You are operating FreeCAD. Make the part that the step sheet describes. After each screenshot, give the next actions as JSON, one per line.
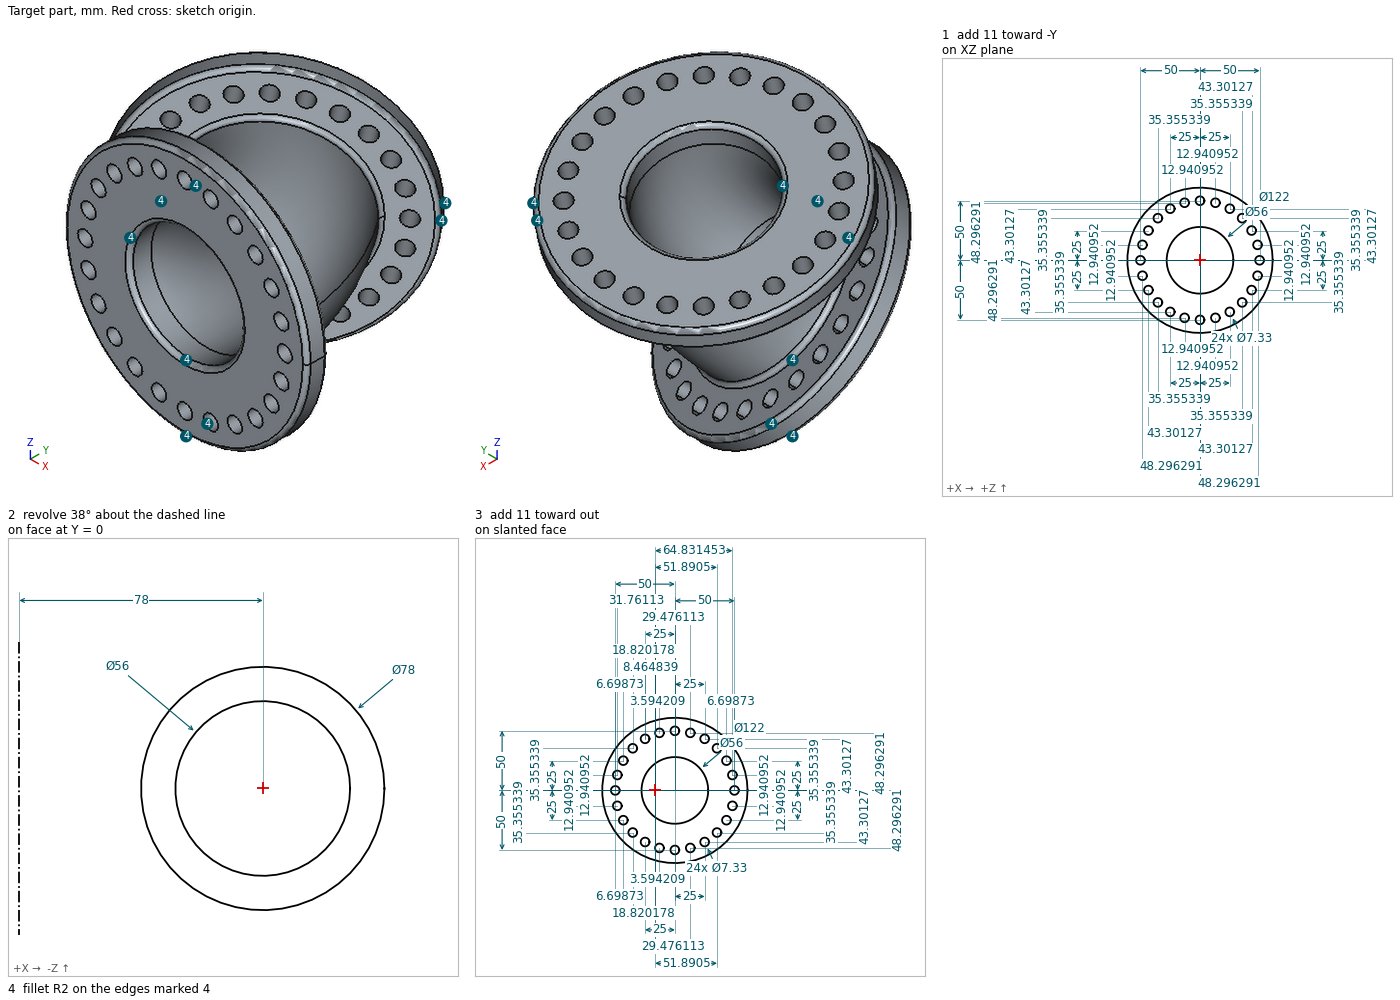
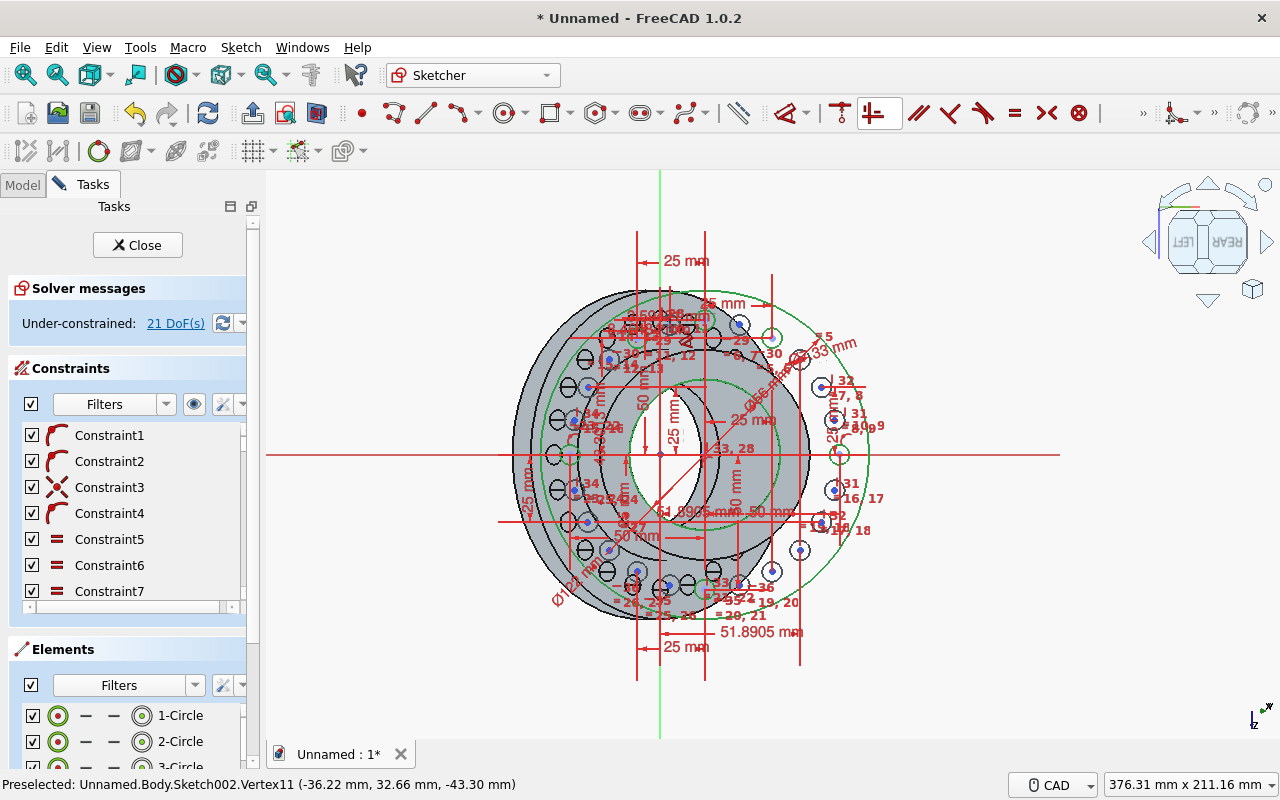
{"action": "left_click", "coordinate": [575, 420]}
{"action": "left_click", "coordinate": [637, 362]}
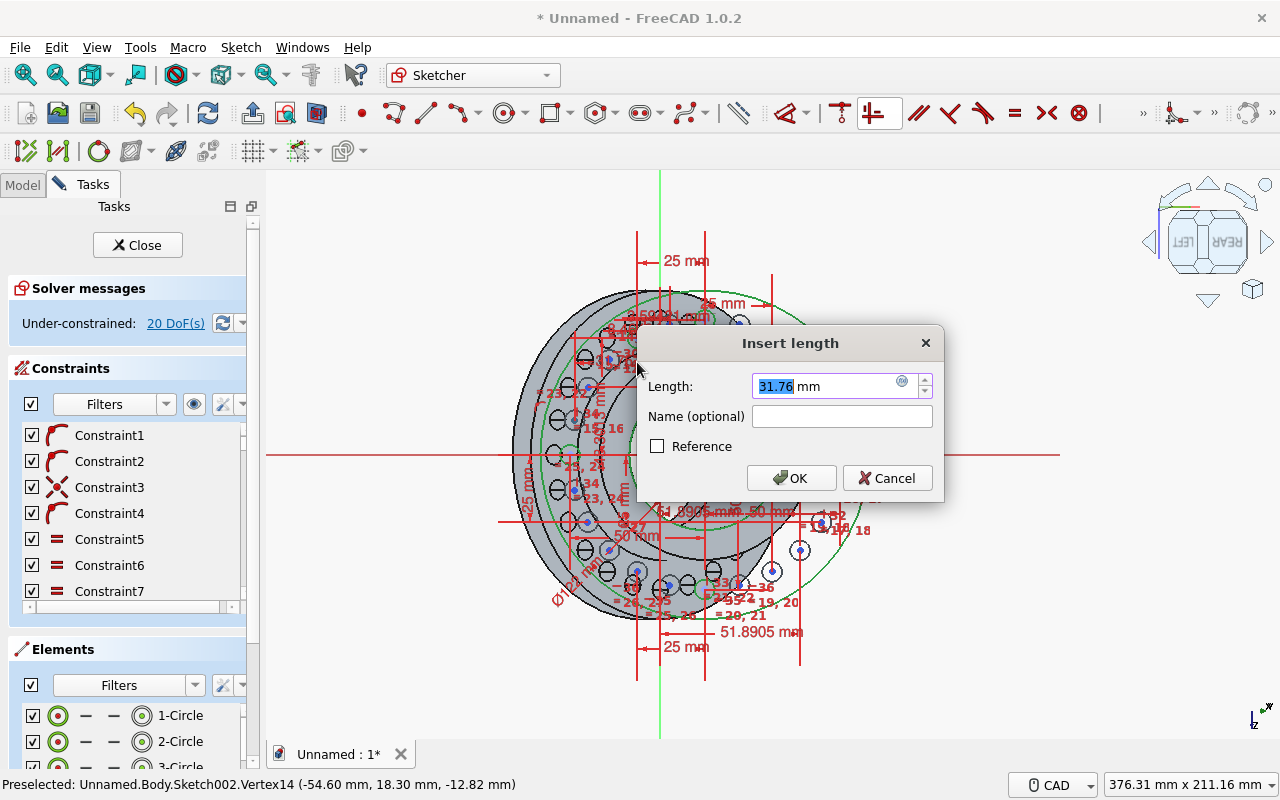
{"action": "type", "text": "31.76113"}
{"action": "key", "text": "Return"}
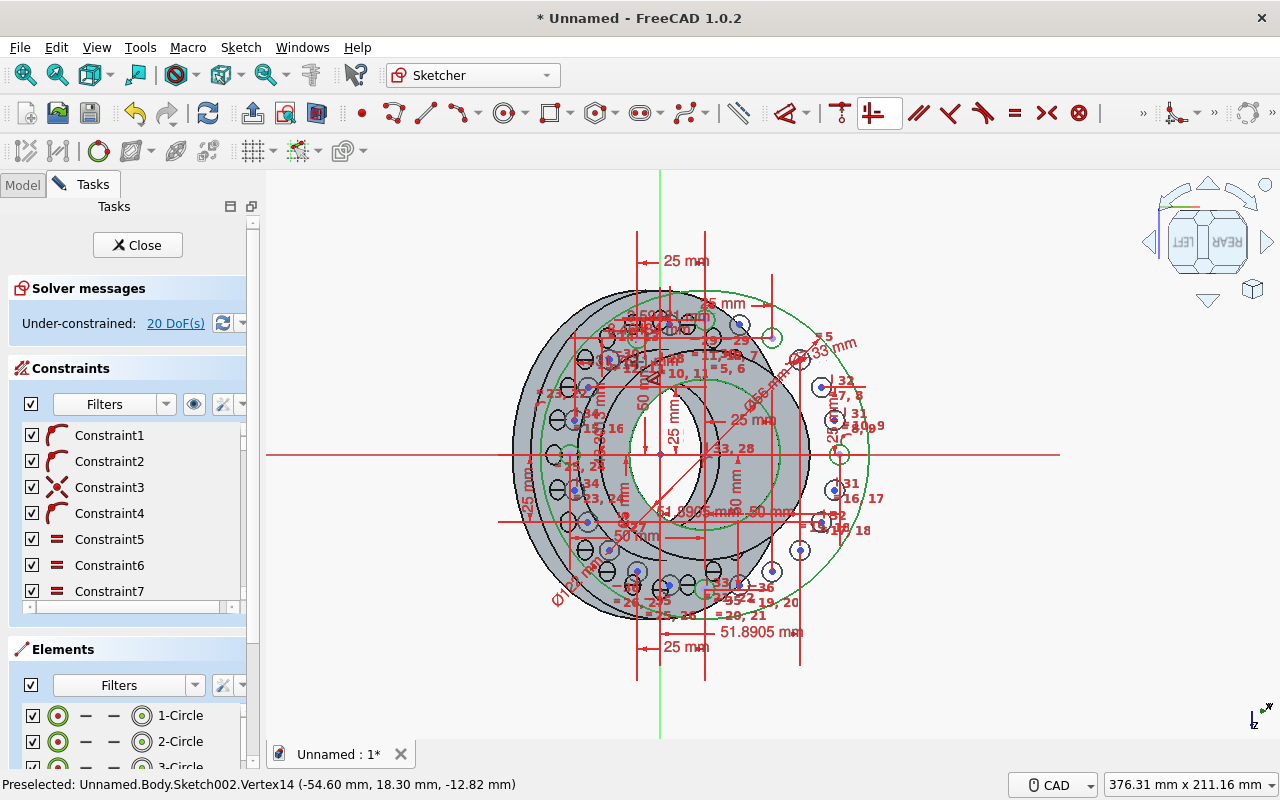
{"action": "left_click", "coordinate": [772, 572]}
{"action": "left_click", "coordinate": [602, 472]}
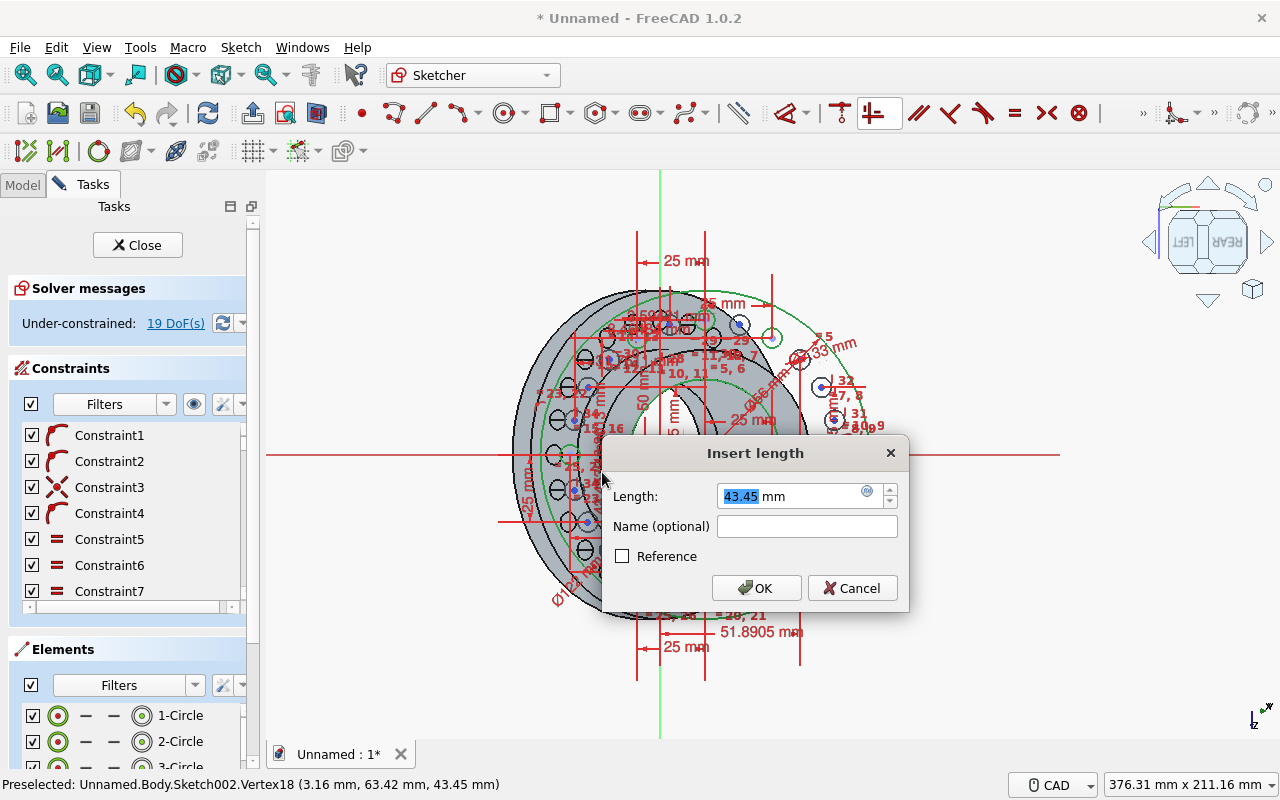
{"action": "type", "text": "43.30127"}
{"action": "key", "text": "Return"}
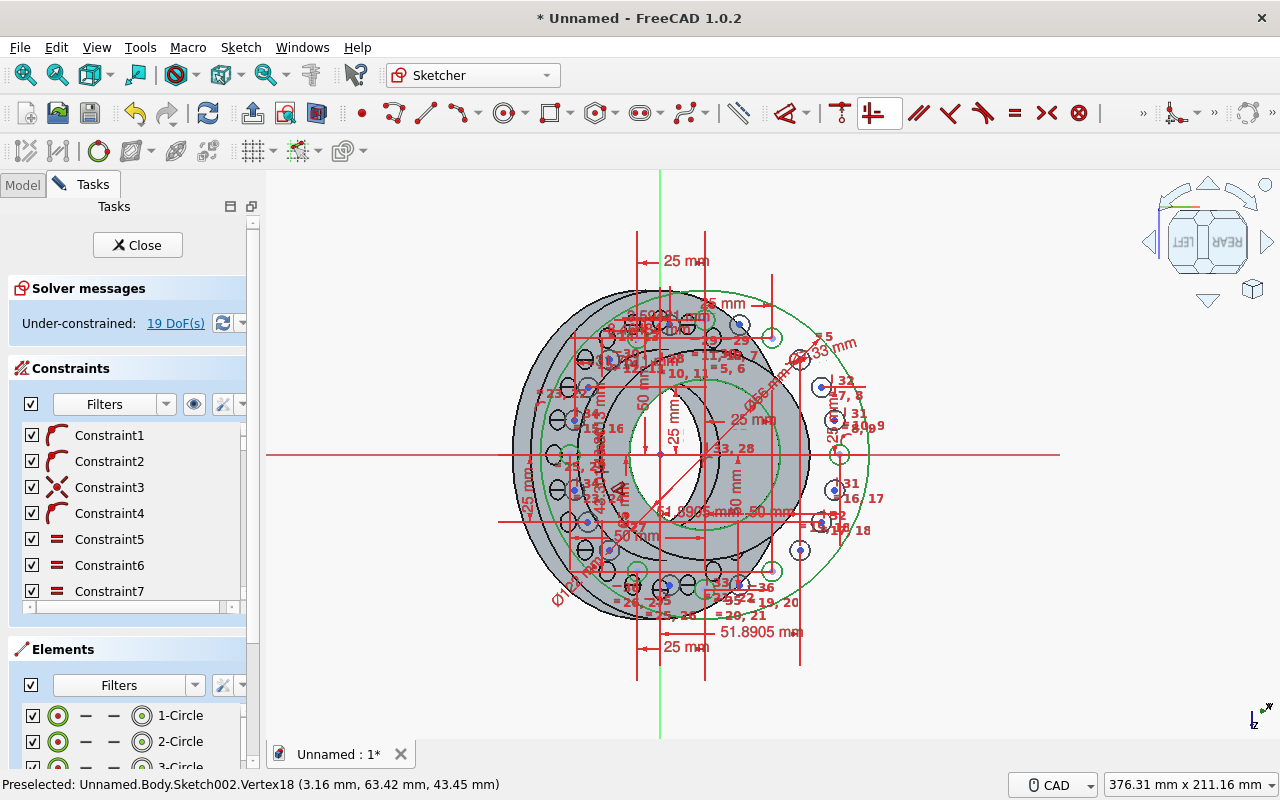
{"action": "scroll", "coordinate": [670, 585], "scroll_direction": "up", "scroll_amount": 8}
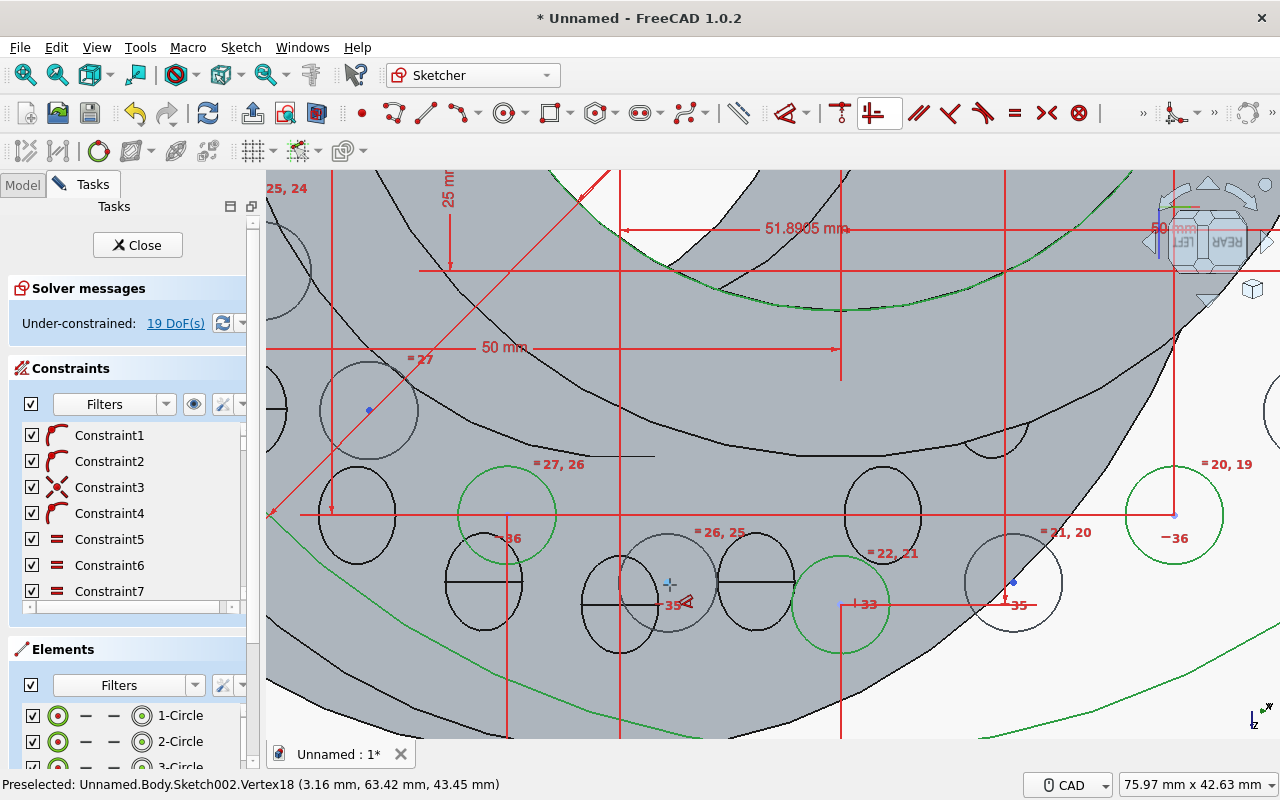
{"action": "left_click", "coordinate": [668, 583]}
{"action": "left_click", "coordinate": [661, 617]}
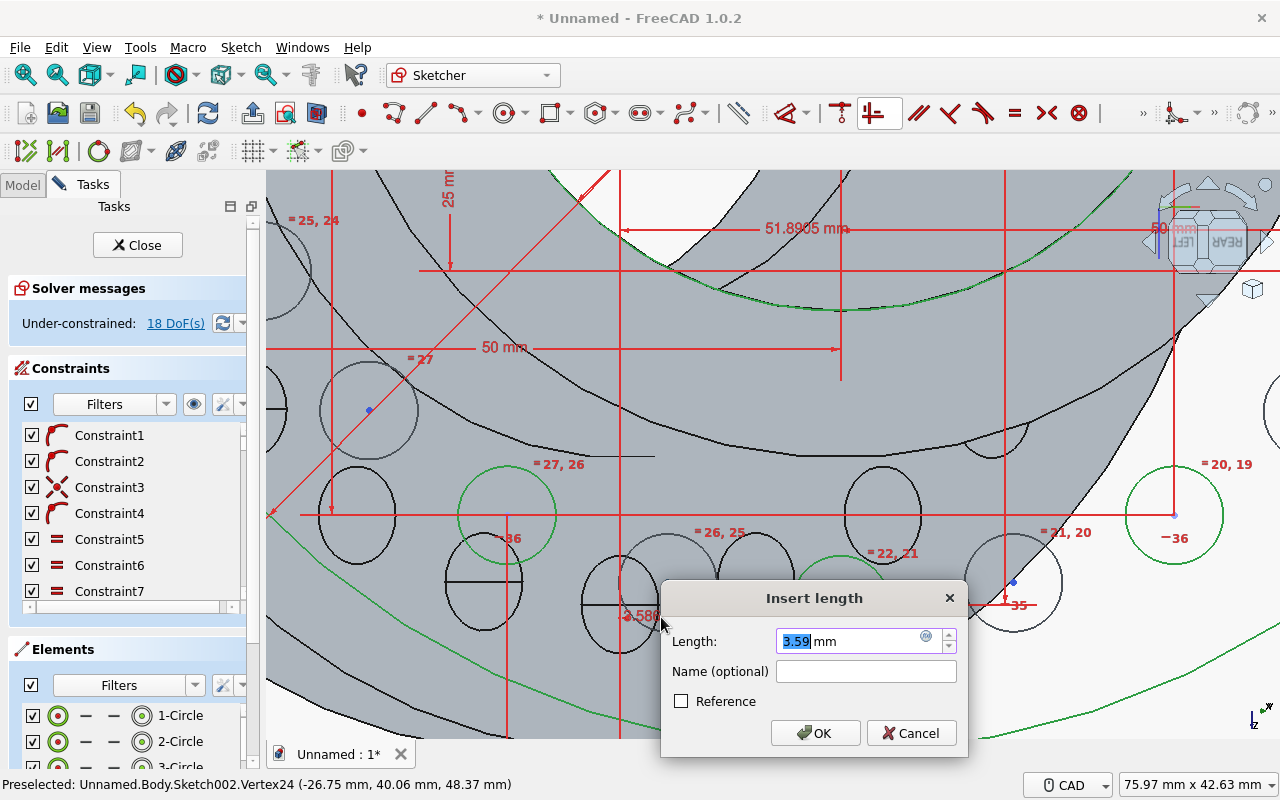
{"action": "type", "text": "3.594209"}
{"action": "key", "text": "Return"}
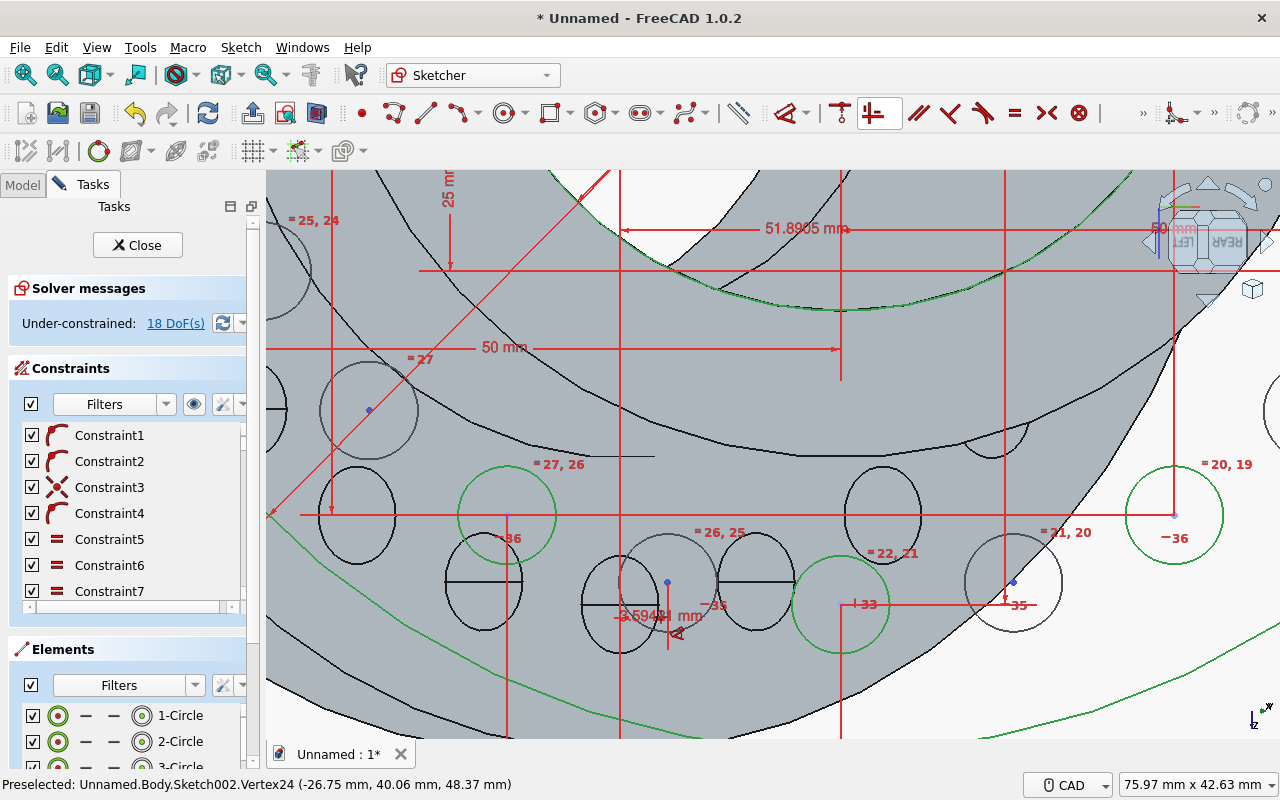
{"action": "scroll", "coordinate": [670, 585], "scroll_direction": "down", "scroll_amount": 8}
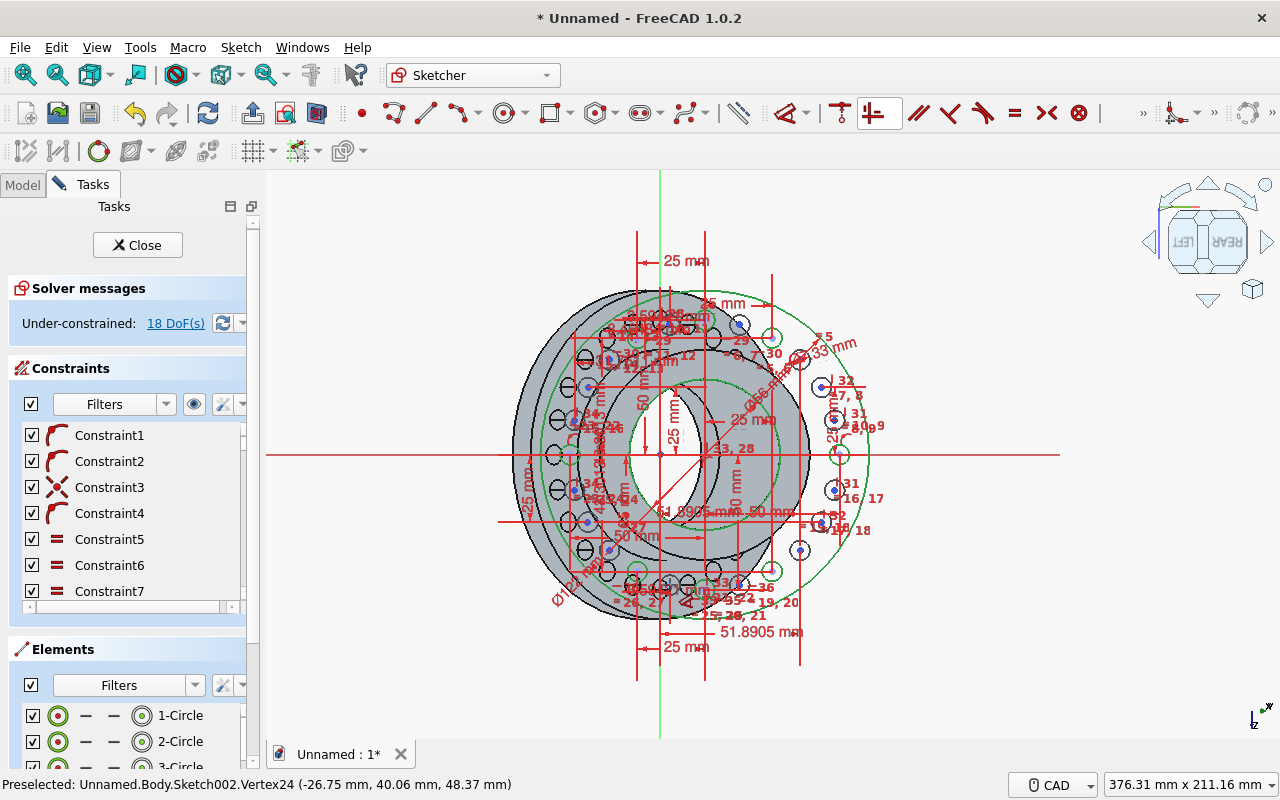
{"action": "scroll", "coordinate": [822, 387], "scroll_direction": "up", "scroll_amount": 4}